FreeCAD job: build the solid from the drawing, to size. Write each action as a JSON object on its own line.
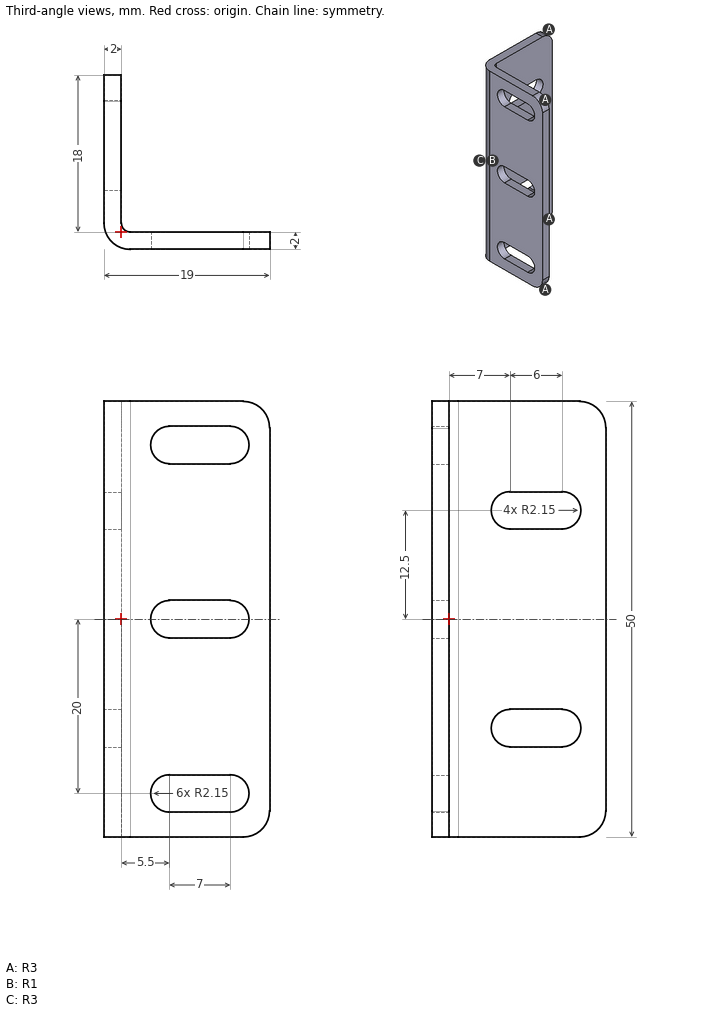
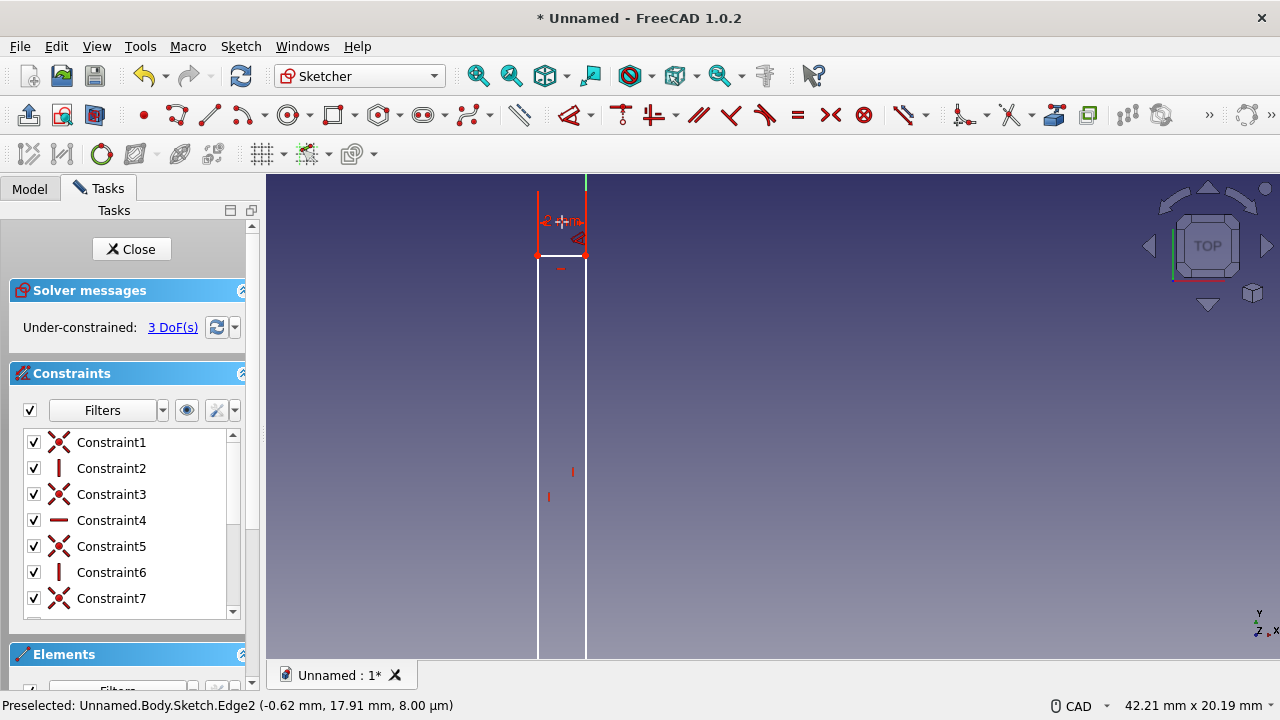
{"action": "scroll", "coordinate": [579, 259], "scroll_direction": "down", "scroll_amount": 2}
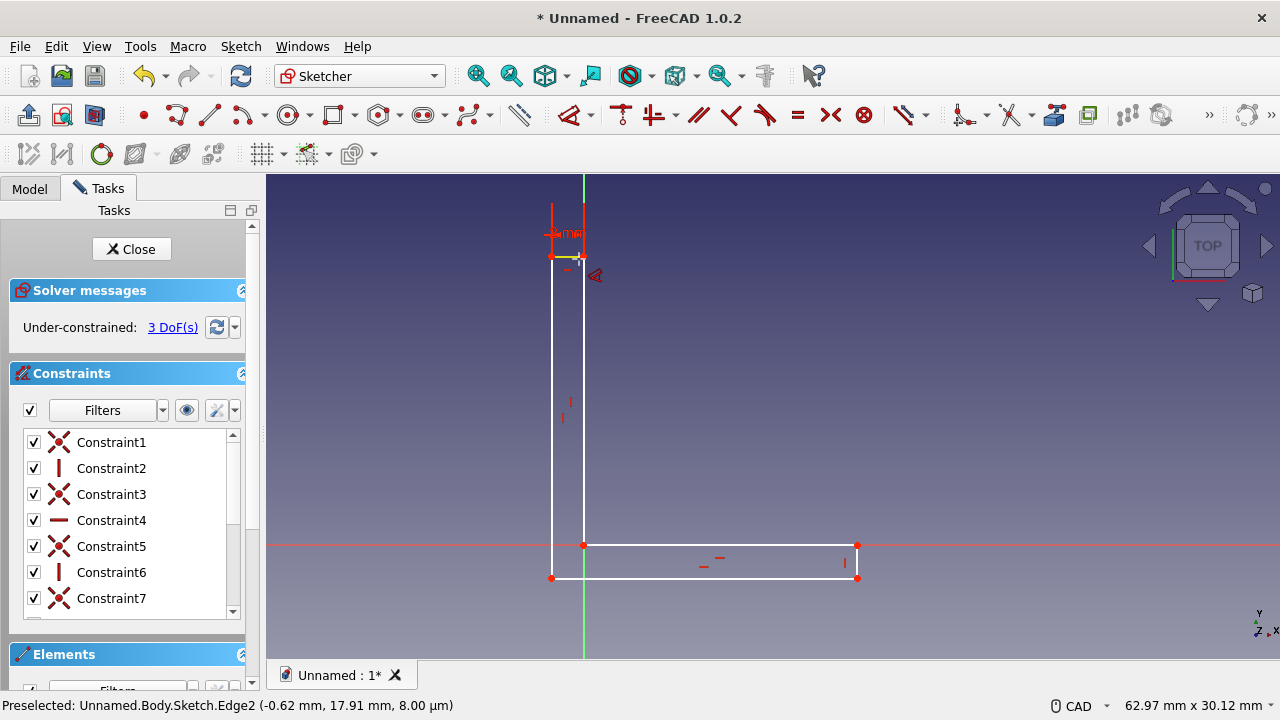
{"action": "scroll", "coordinate": [857, 569], "scroll_direction": "up", "scroll_amount": 2}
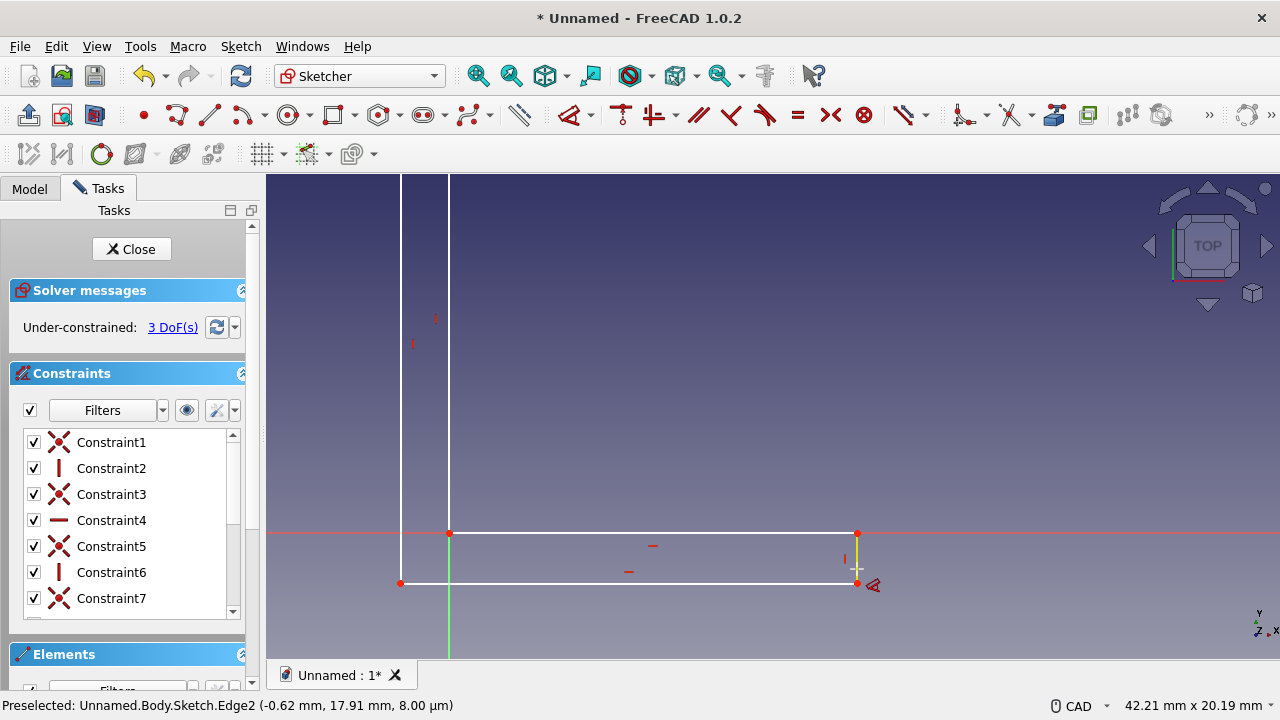
{"action": "left_click", "coordinate": [857, 568]}
{"action": "left_click", "coordinate": [891, 558]}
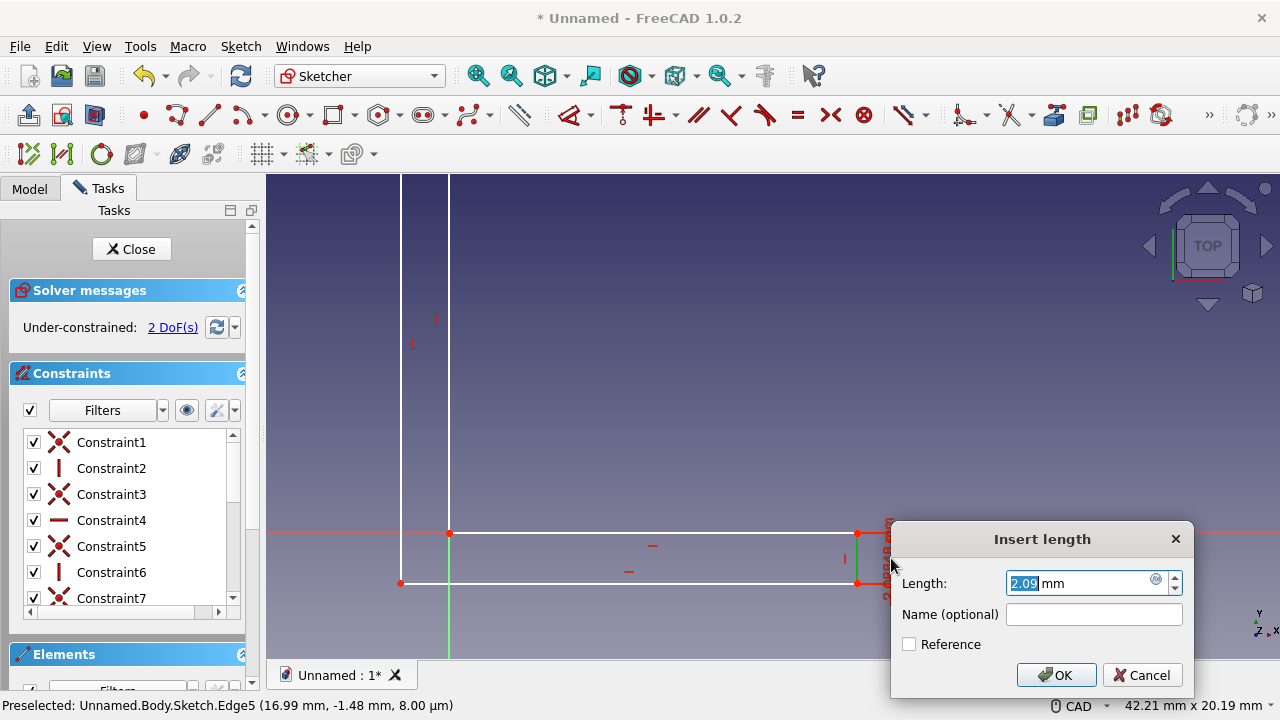
{"action": "type", "text": "2"}
{"action": "key", "text": "Return"}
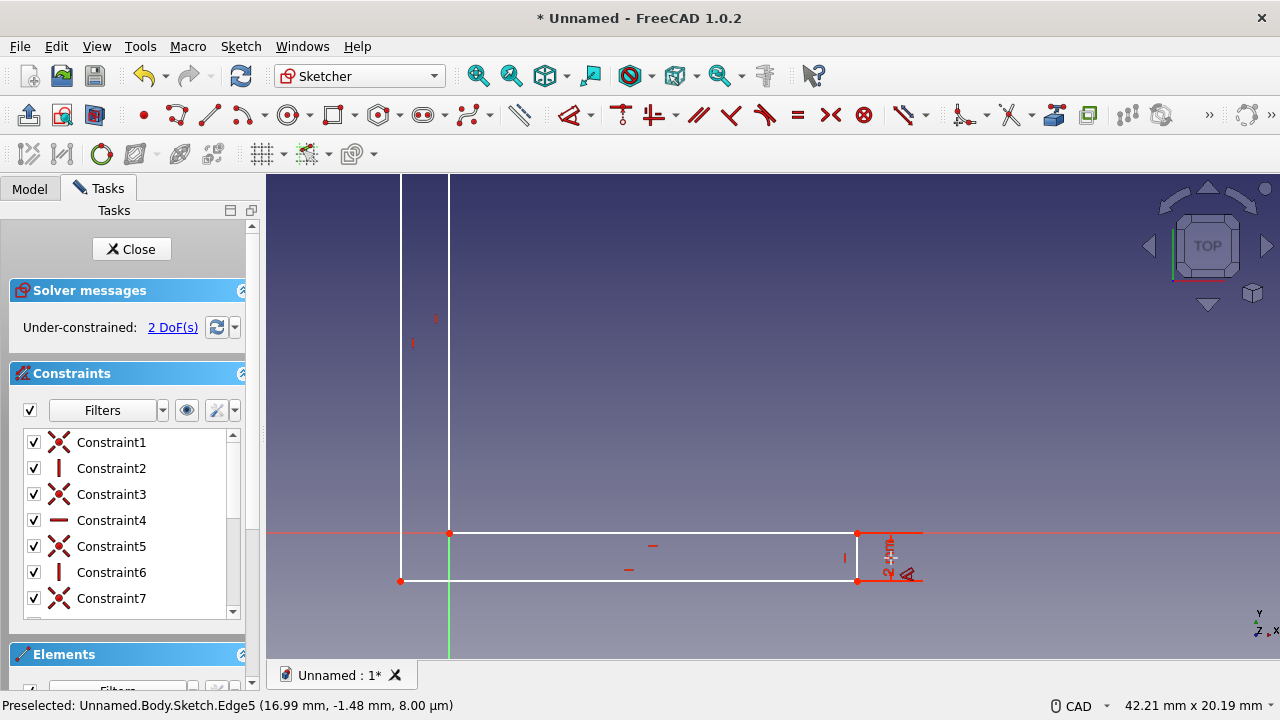
{"action": "left_click", "coordinate": [449, 404]}
{"action": "left_click", "coordinate": [415, 368]}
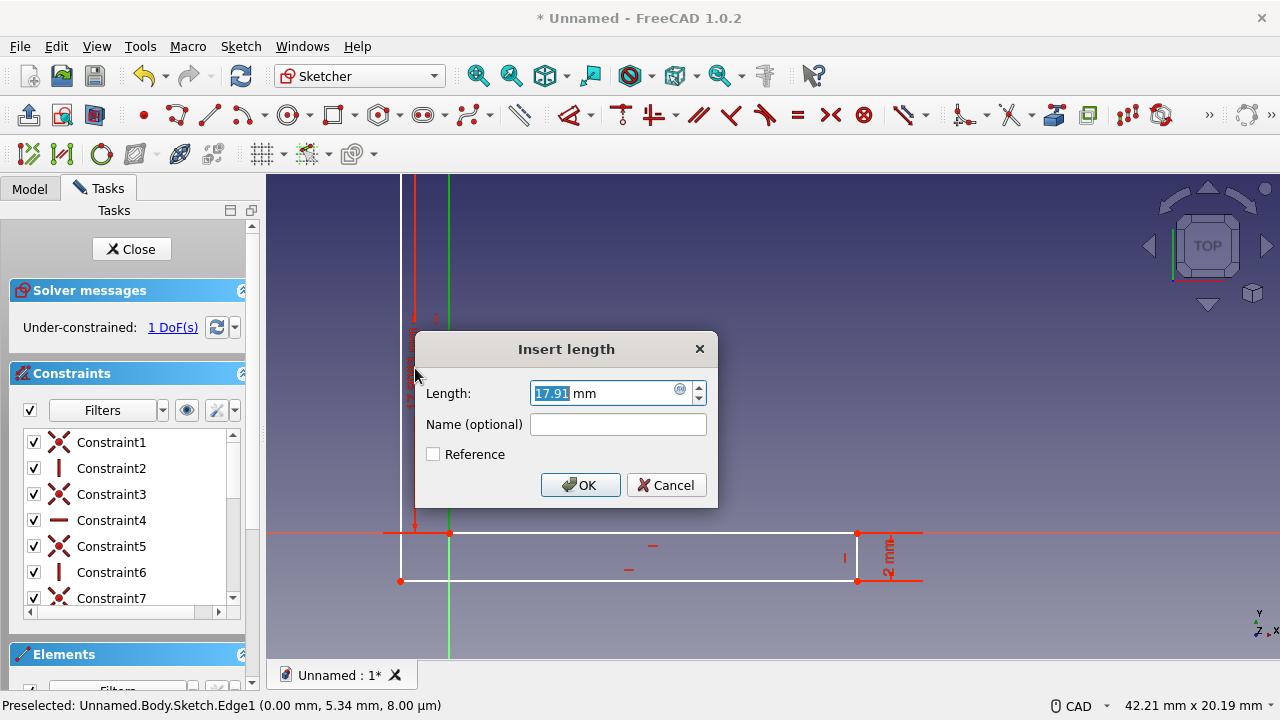
{"action": "type", "text": "18"}
{"action": "key", "text": "Return"}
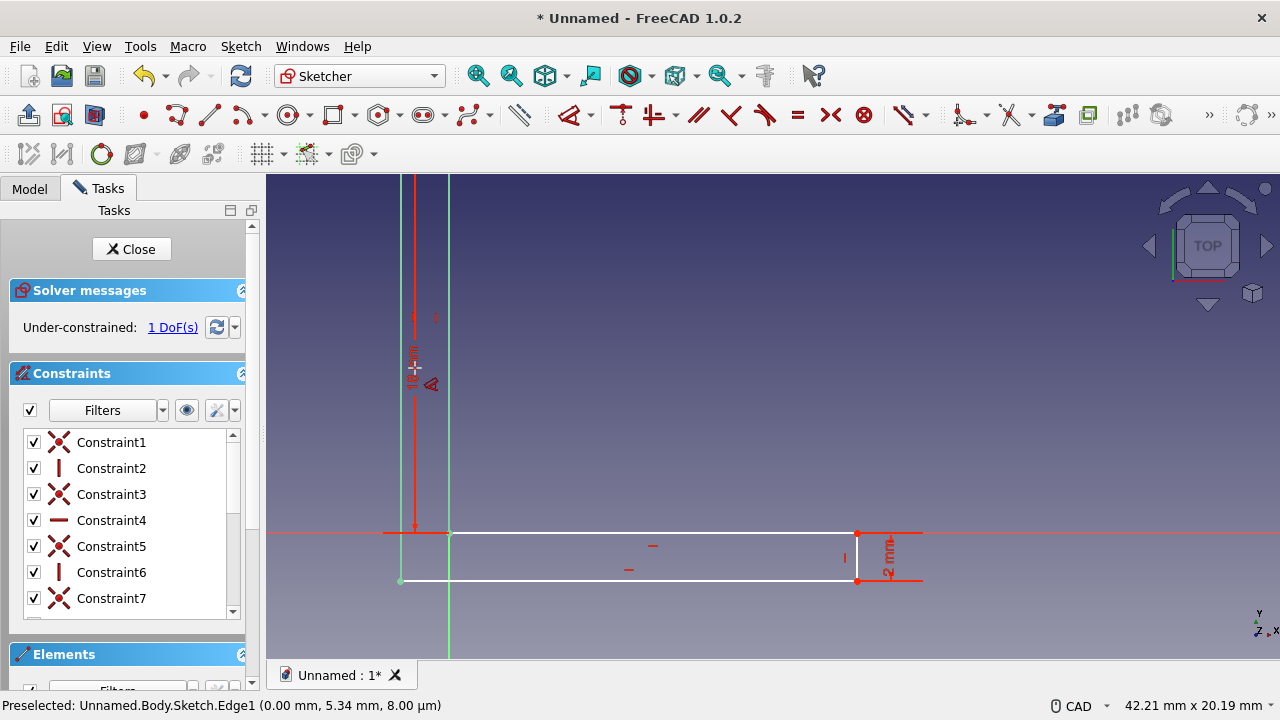
{"action": "left_click", "coordinate": [538, 581]}
{"action": "left_click", "coordinate": [629, 615]}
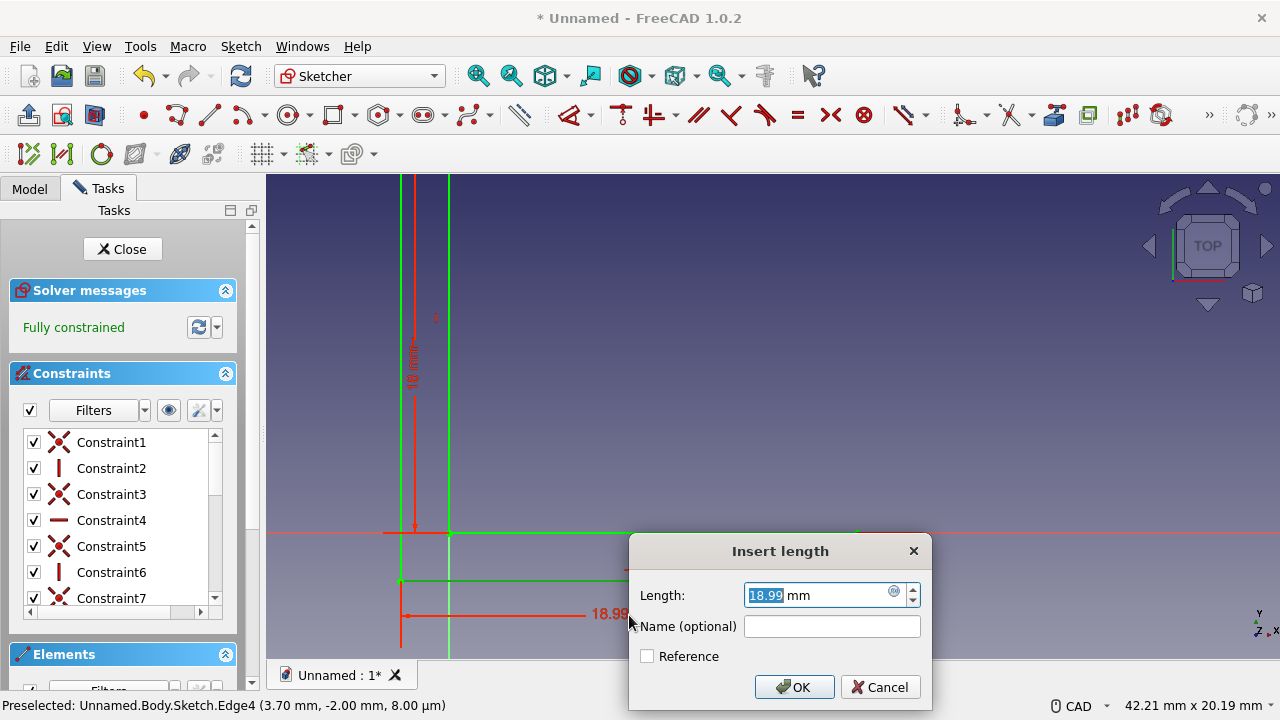
{"action": "type", "text": "19"}
{"action": "key", "text": "Return"}
{"action": "key", "text": "Escape"}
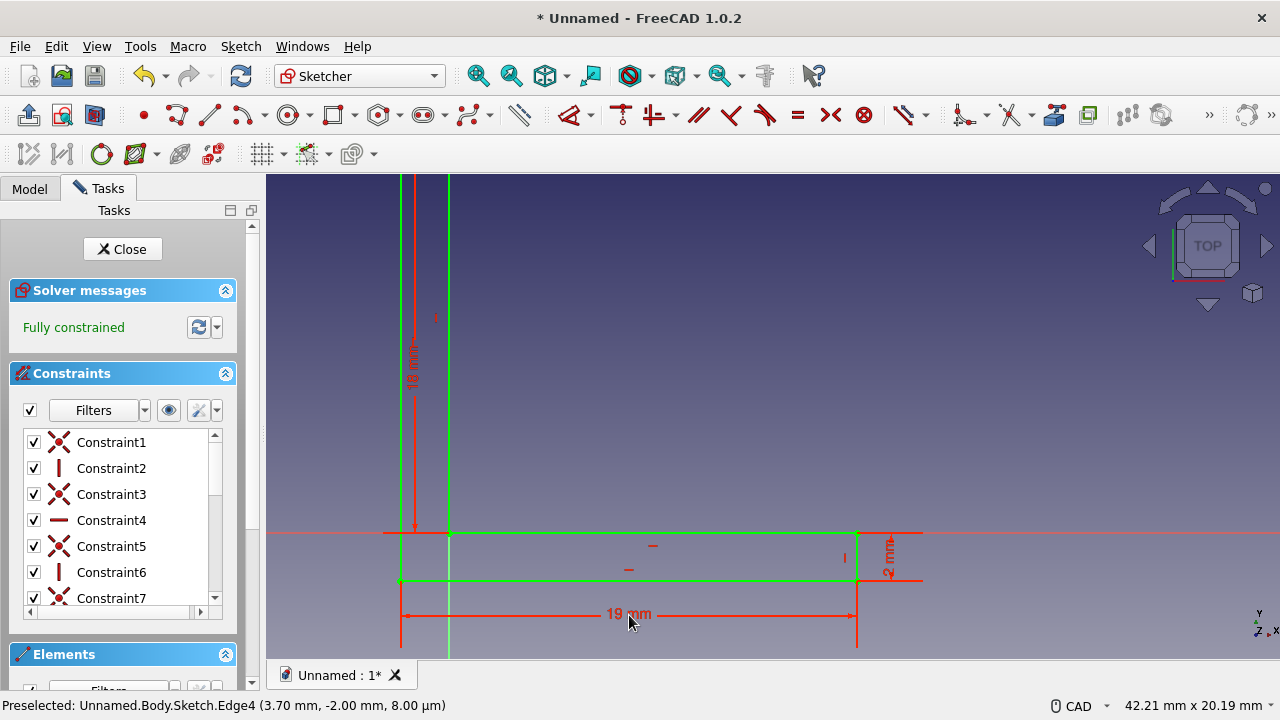
{"action": "left_click", "coordinate": [123, 249]}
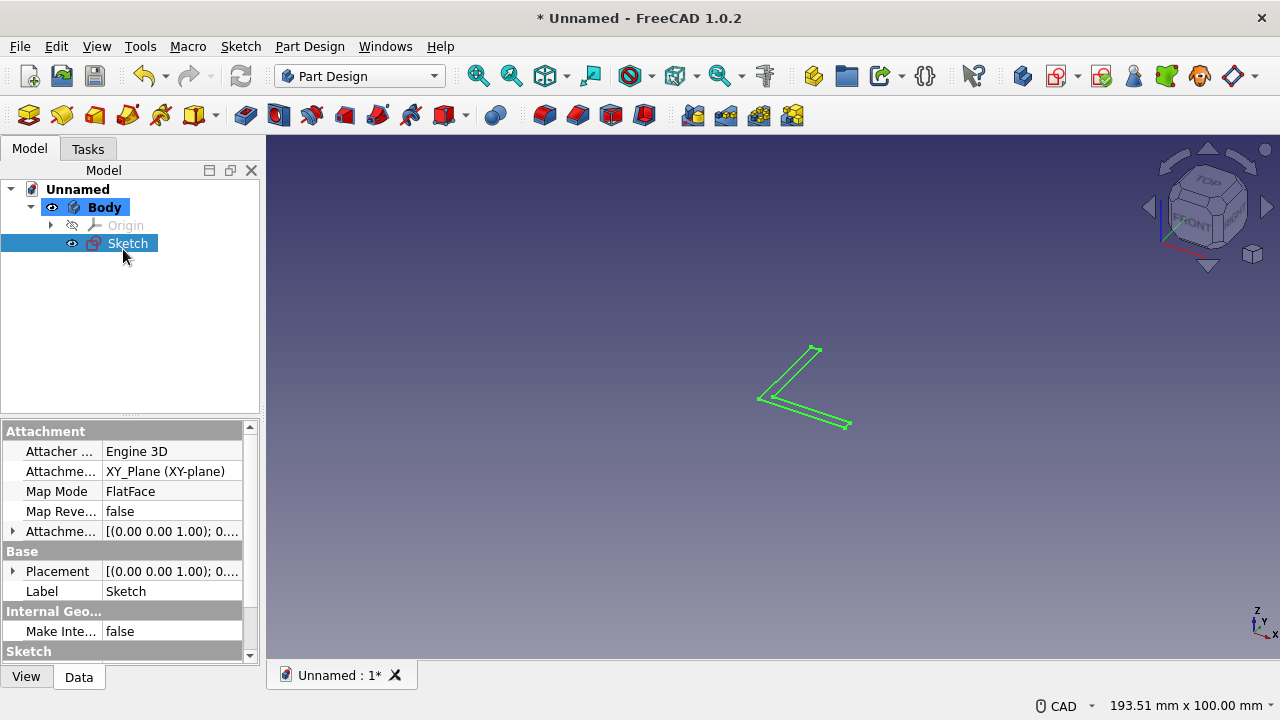
{"action": "left_click", "coordinate": [29, 116]}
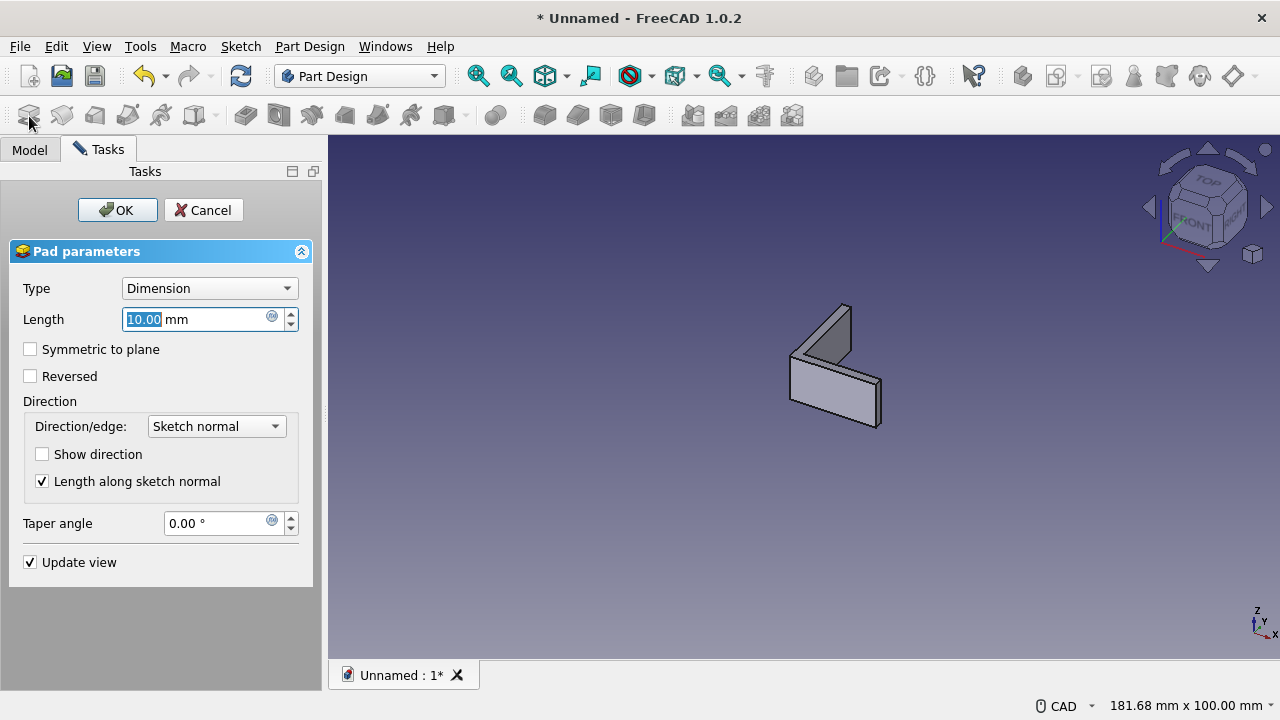
{"action": "type", "text": "50"}
{"action": "key", "text": "Tab"}